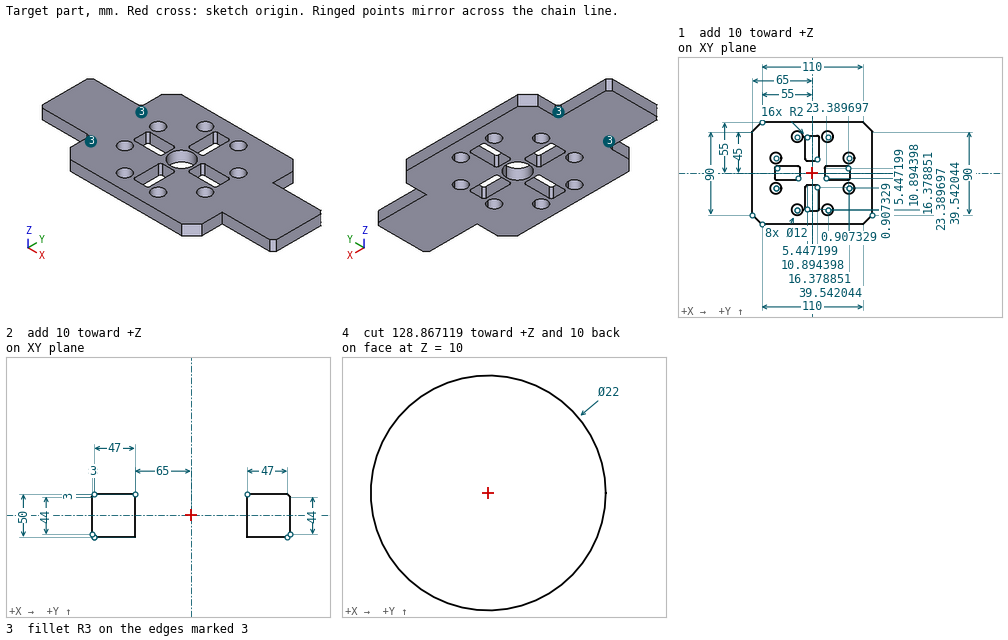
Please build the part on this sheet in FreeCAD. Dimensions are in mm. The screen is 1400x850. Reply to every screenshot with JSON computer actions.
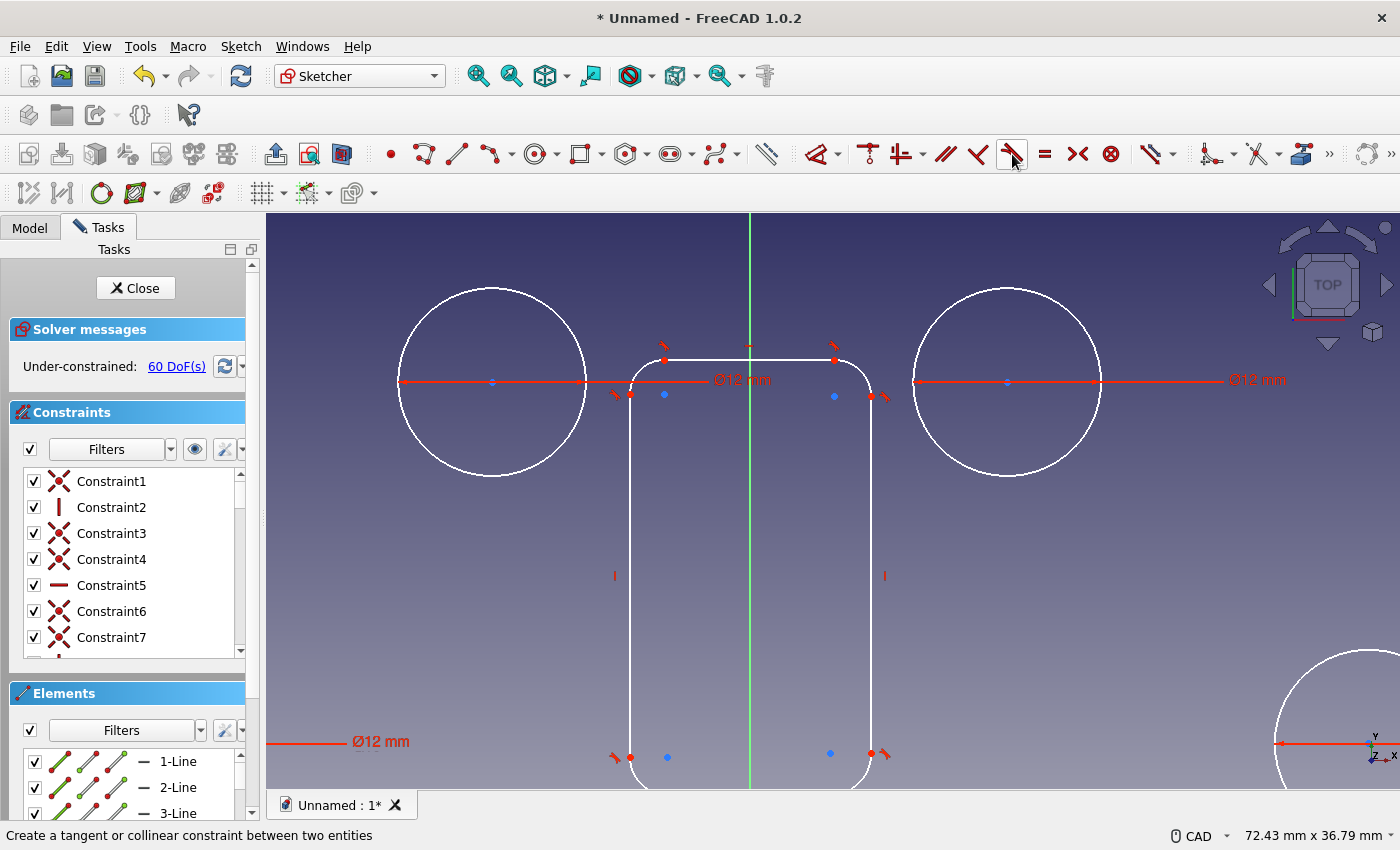
{"action": "scroll", "coordinate": [768, 376], "scroll_direction": "down", "scroll_amount": 8}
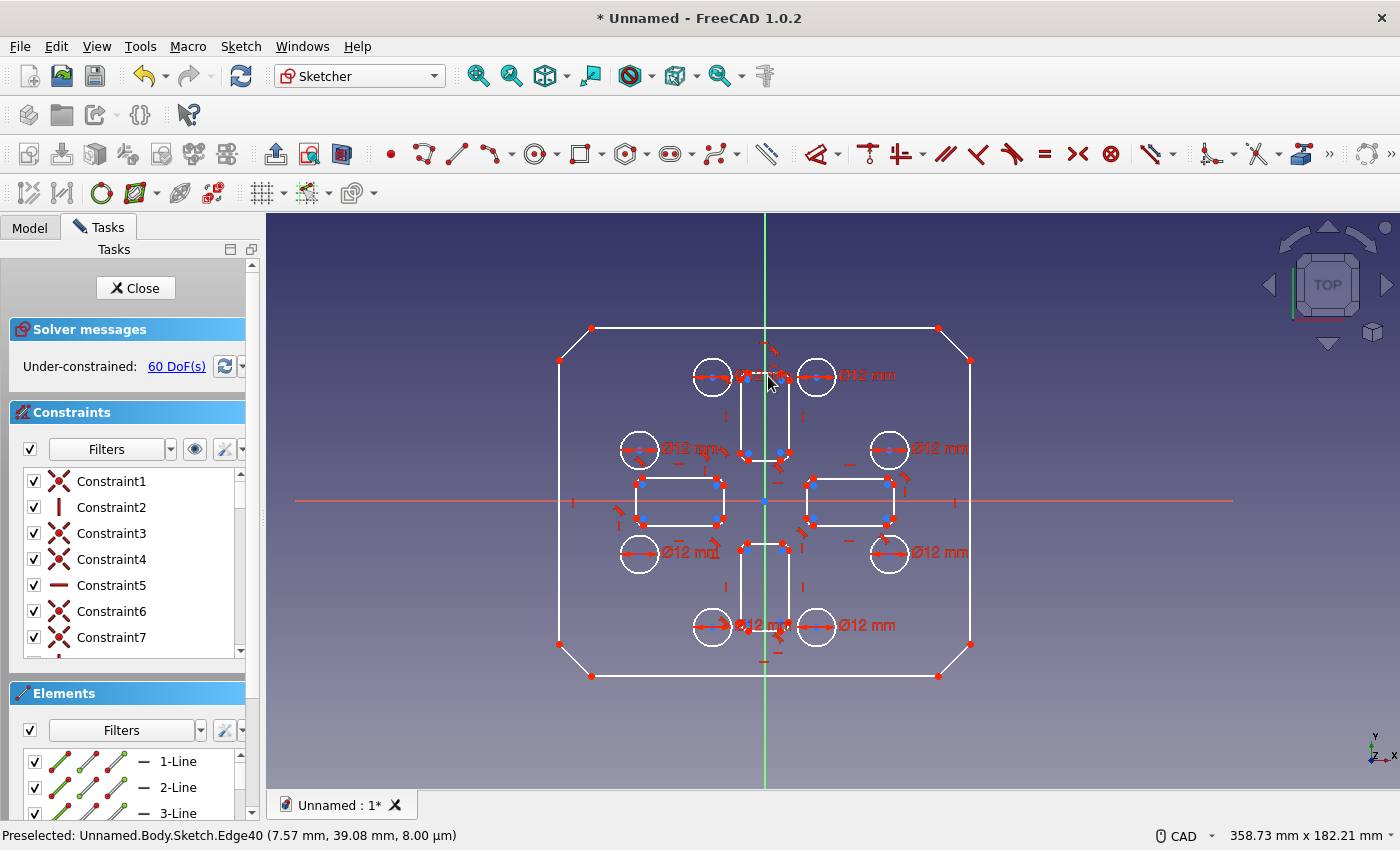
{"action": "scroll", "coordinate": [788, 547], "scroll_direction": "up", "scroll_amount": 8}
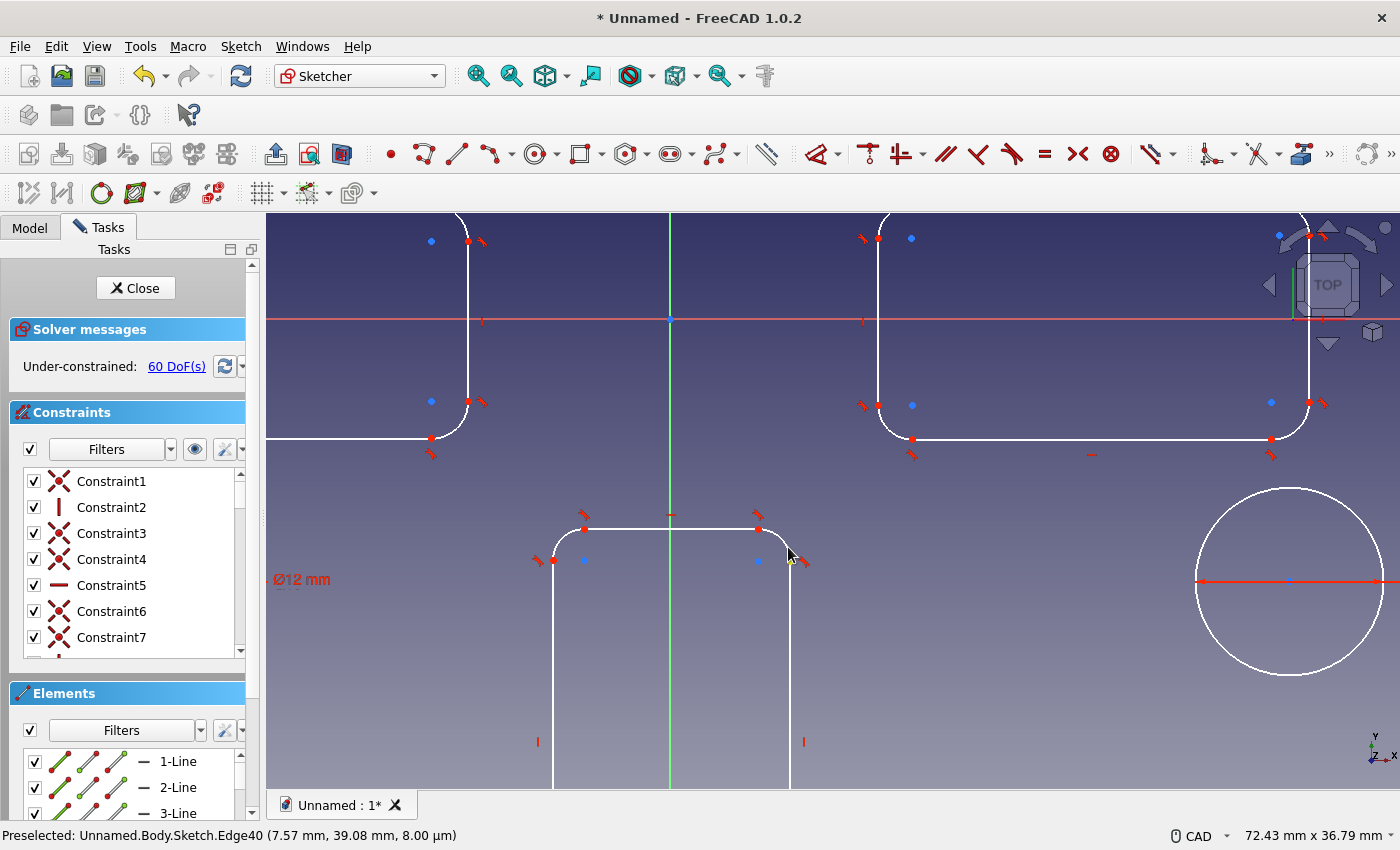
{"action": "left_click", "coordinate": [787, 547]}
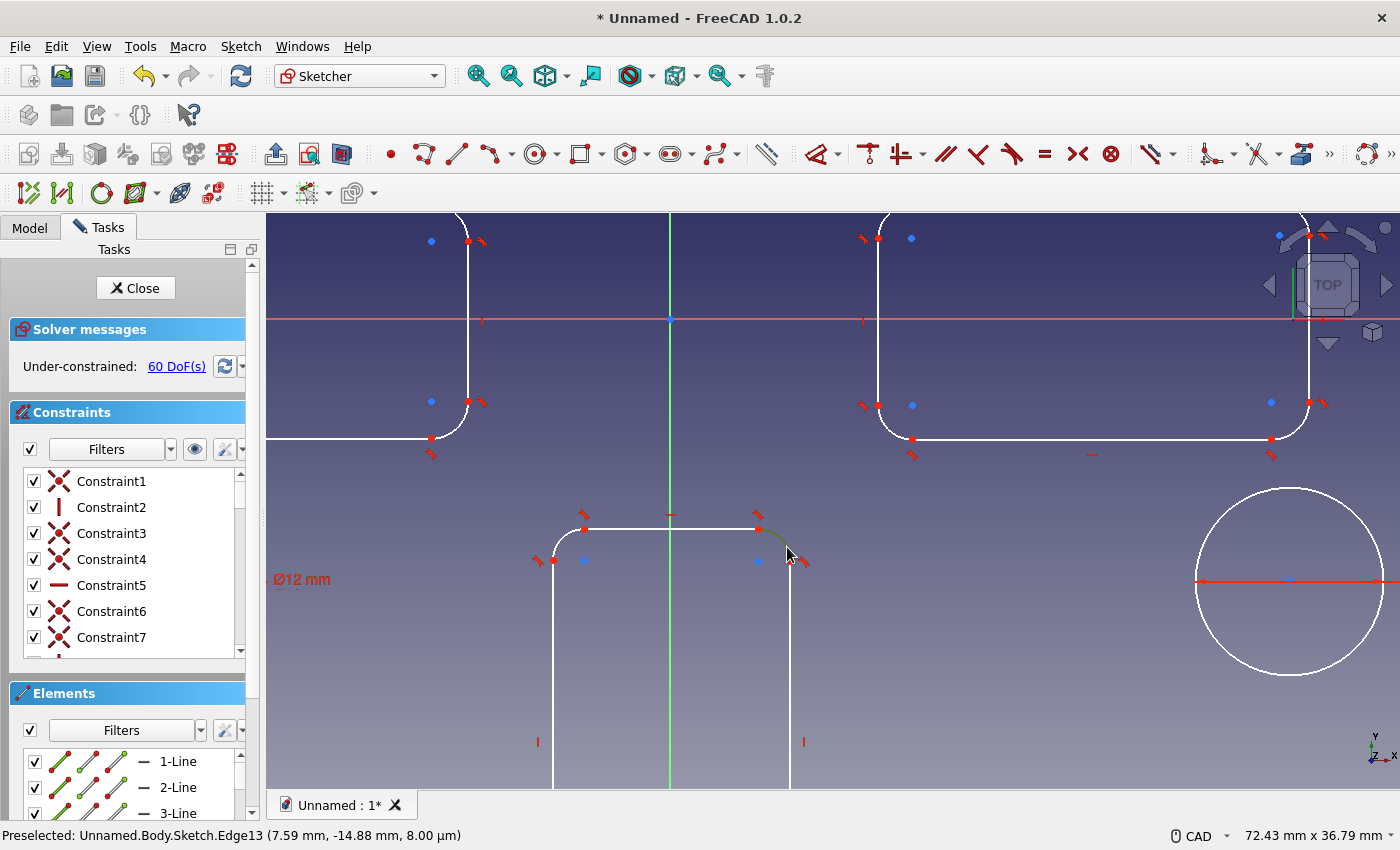
{"action": "scroll", "coordinate": [788, 547], "scroll_direction": "down", "scroll_amount": 8}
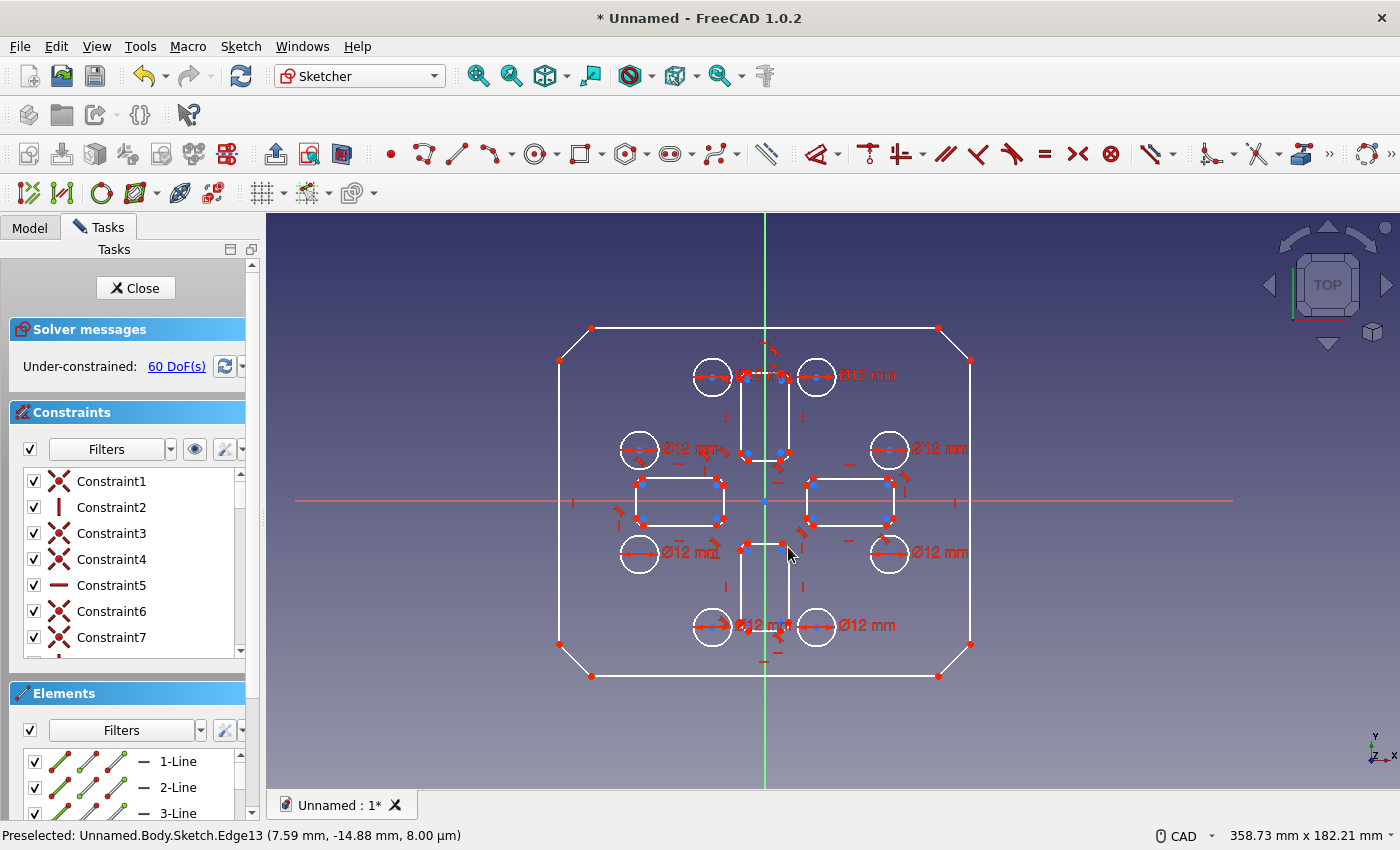
{"action": "scroll", "coordinate": [784, 630], "scroll_direction": "up", "scroll_amount": 7}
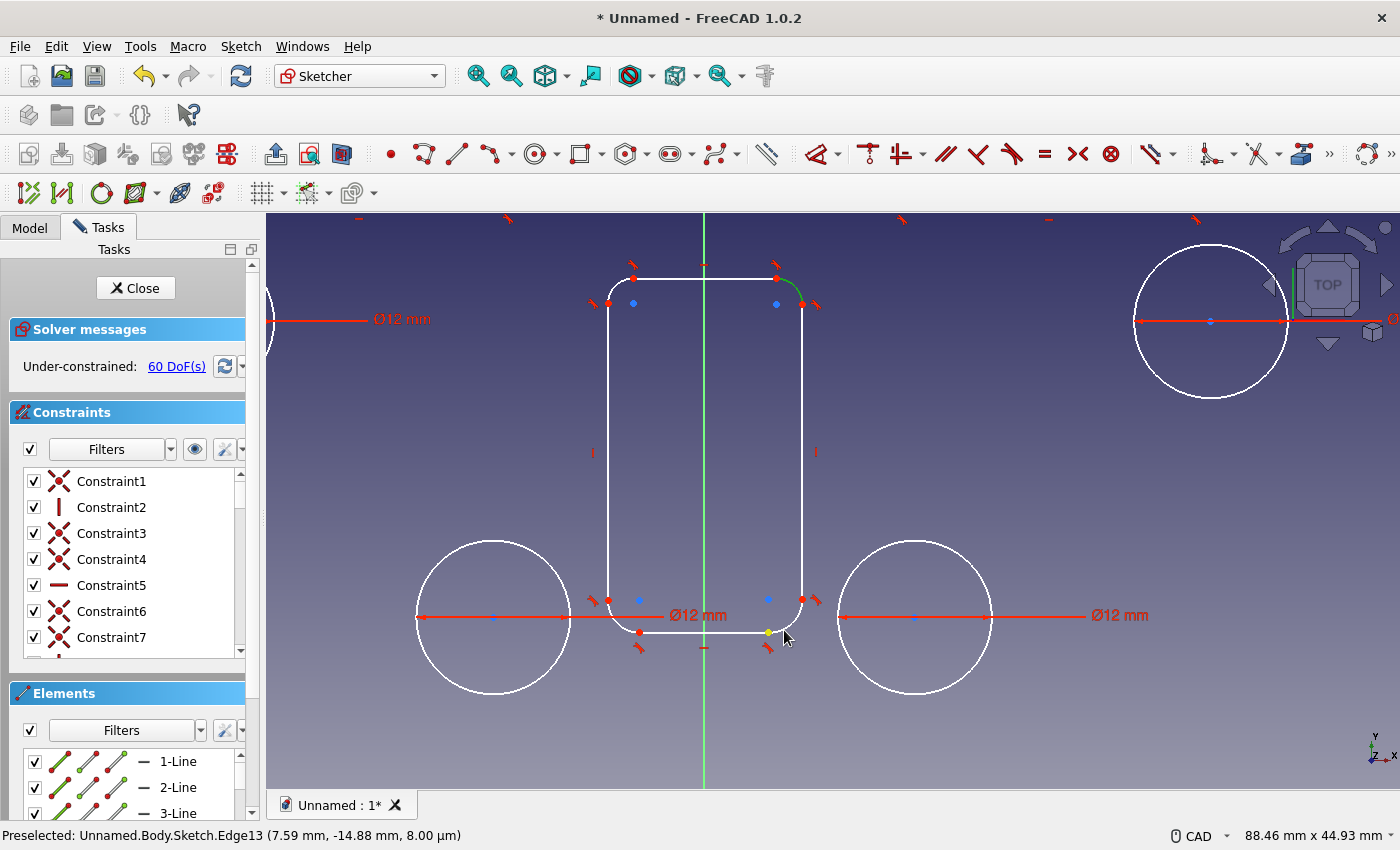
{"action": "left_click", "coordinate": [784, 629]}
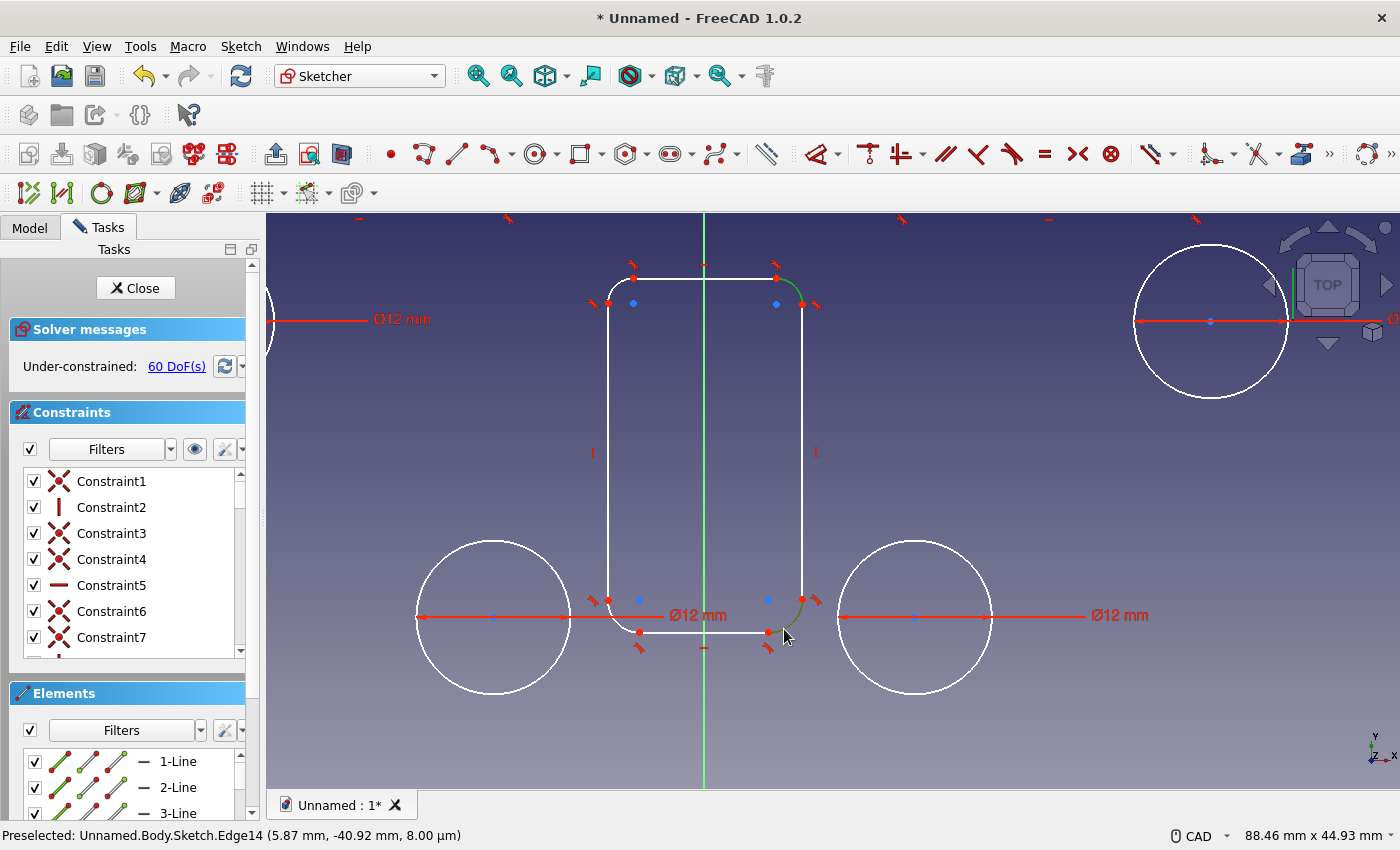
{"action": "left_click", "coordinate": [612, 615]}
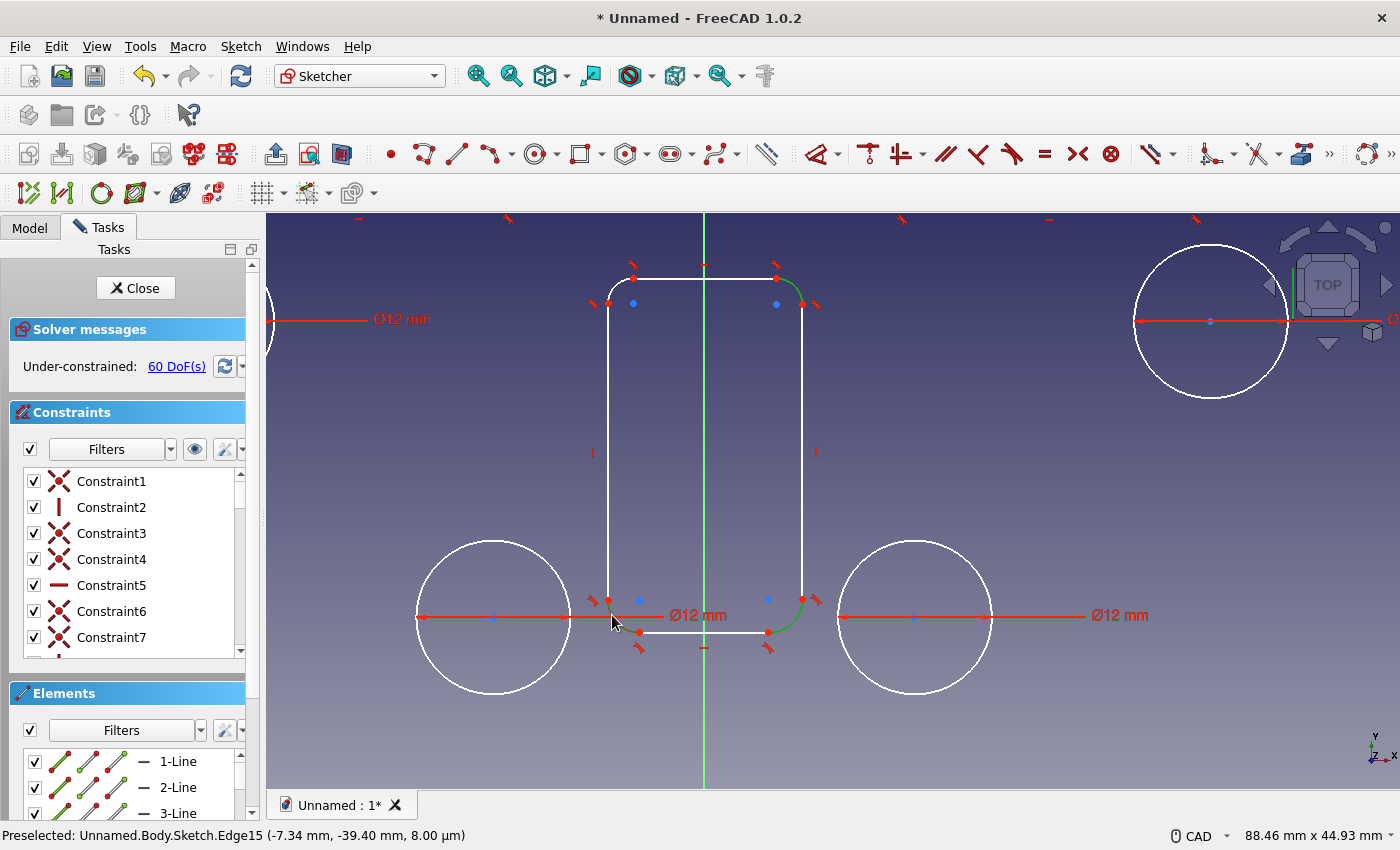
{"action": "left_click", "coordinate": [622, 281]}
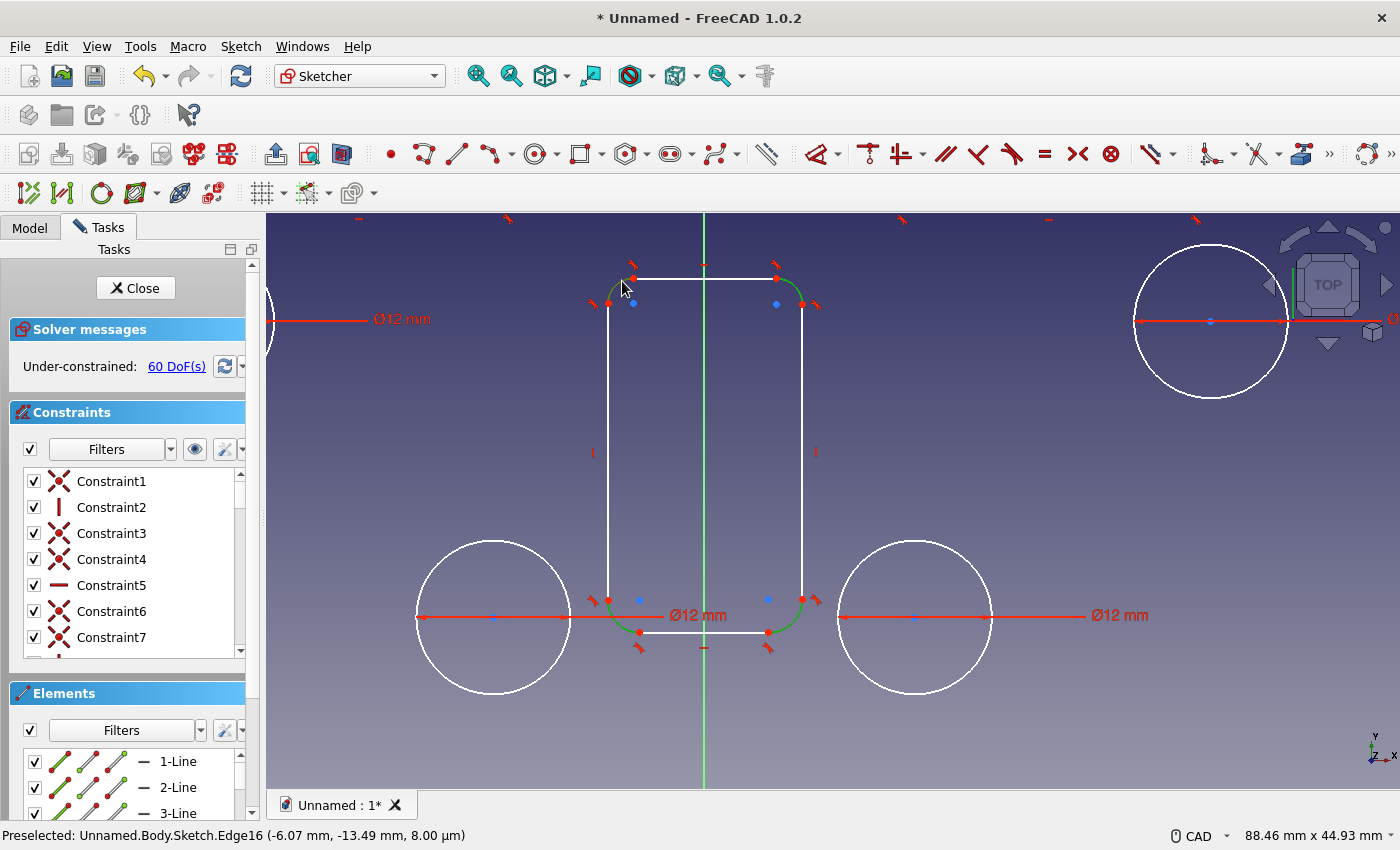
{"action": "scroll", "coordinate": [784, 630], "scroll_direction": "down", "scroll_amount": 7}